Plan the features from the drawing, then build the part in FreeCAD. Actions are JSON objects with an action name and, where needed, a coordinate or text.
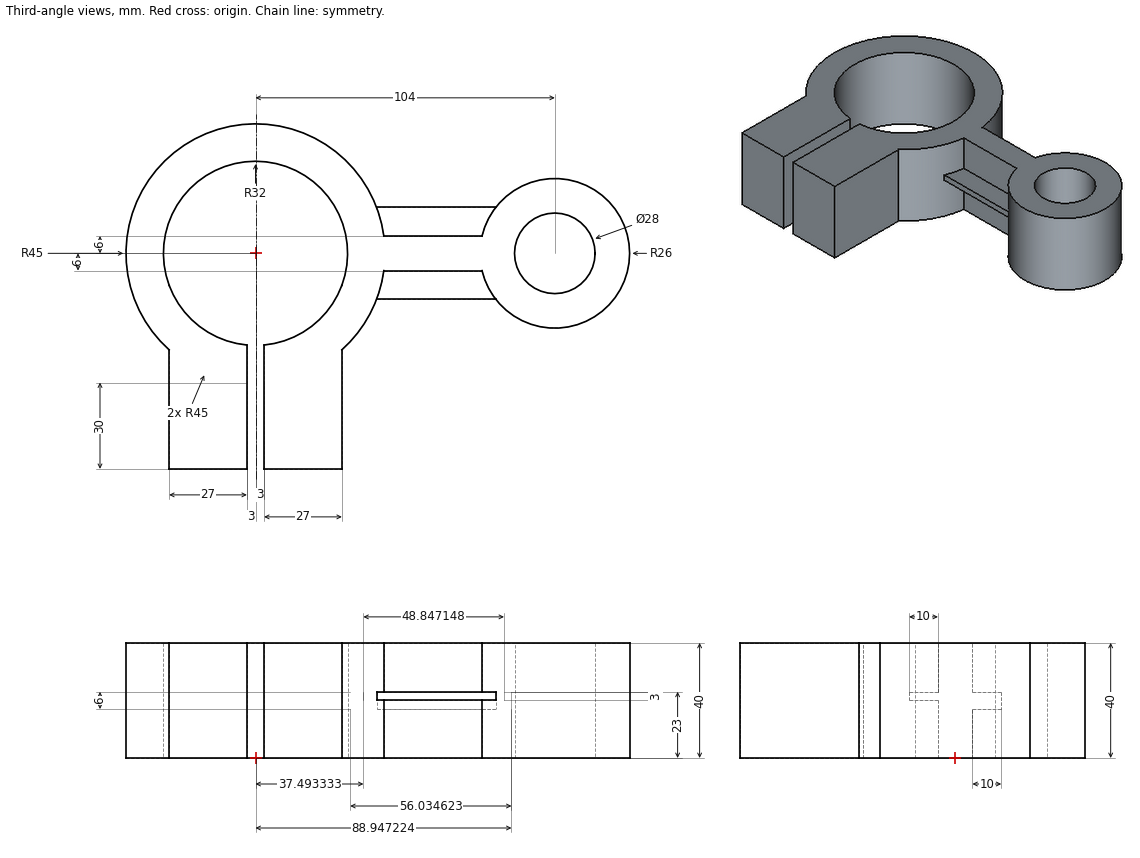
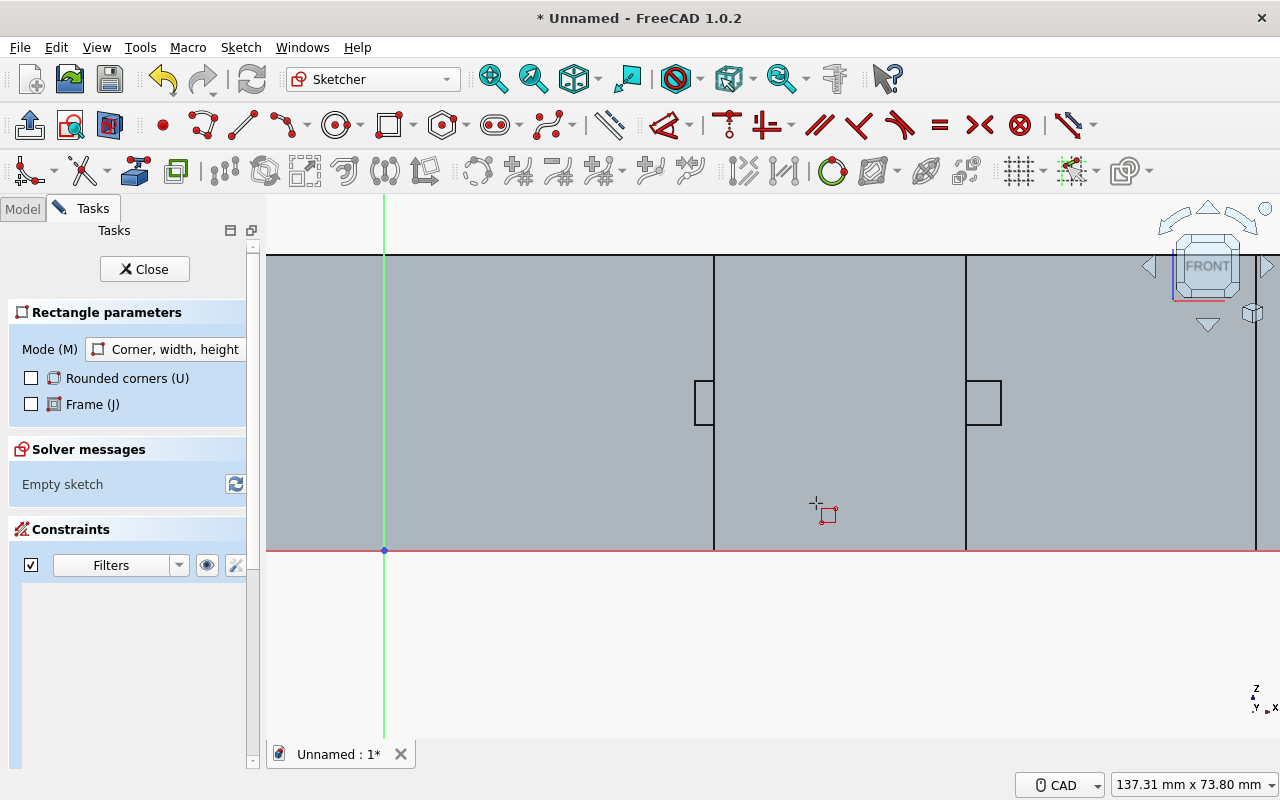
{"action": "left_click", "coordinate": [661, 381]}
{"action": "mouse_move", "coordinate": [1022, 403]}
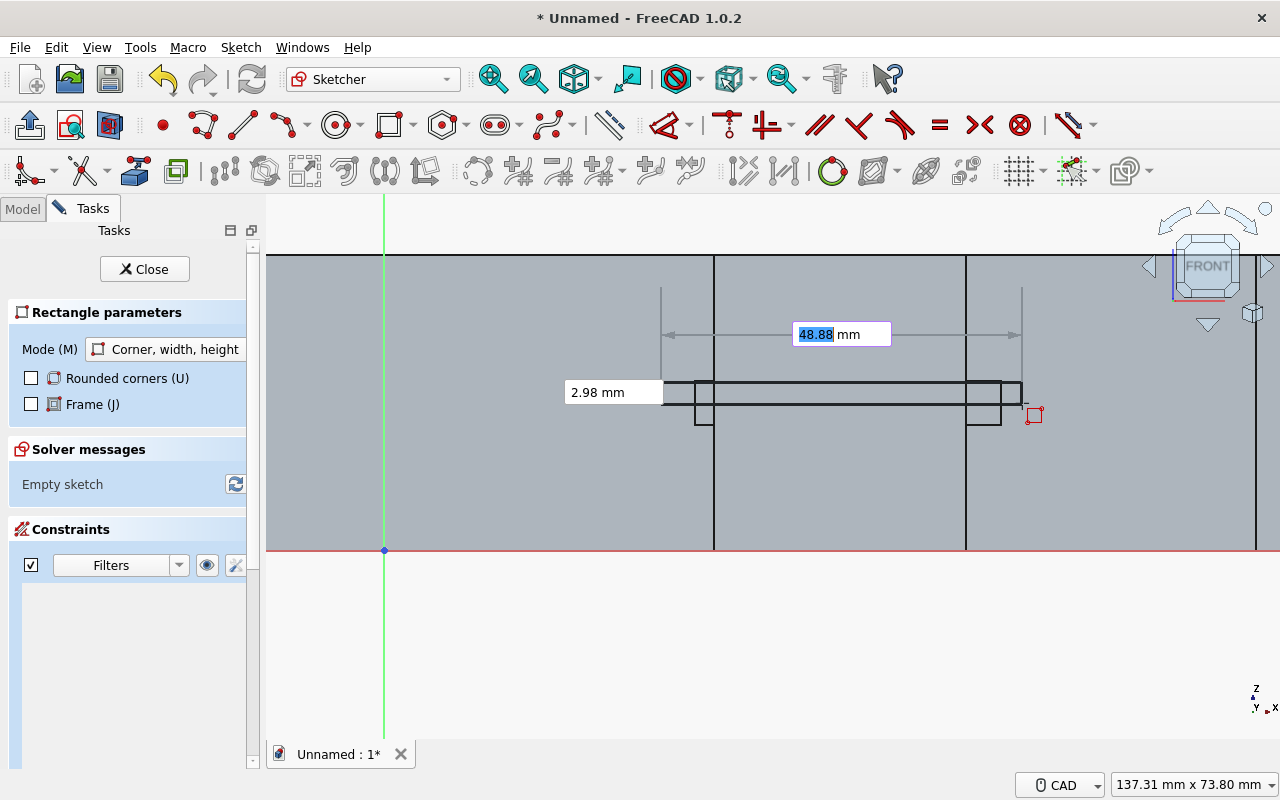
{"action": "type", "text": "48.847148"}
{"action": "key", "text": "Tab"}
{"action": "type", "text": "3"}
{"action": "key", "text": "Return"}
{"action": "key", "text": "Escape"}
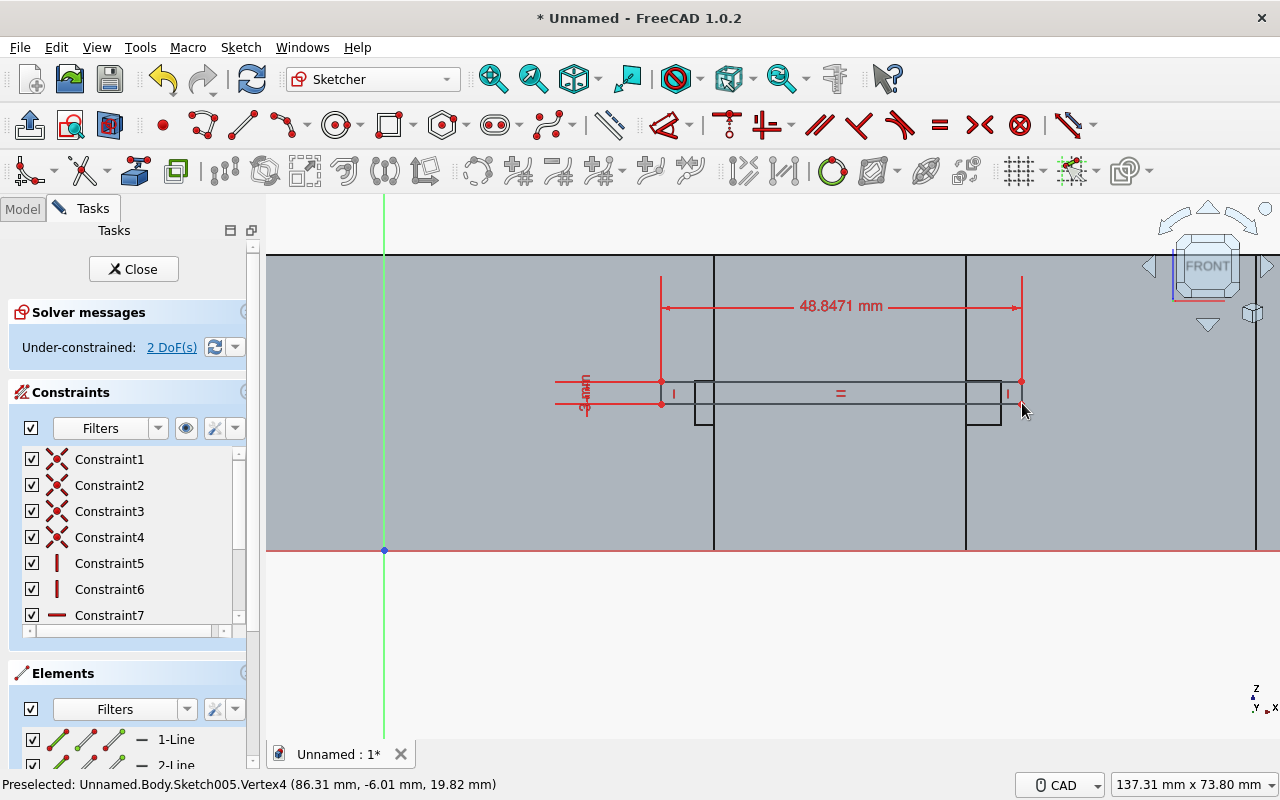
{"action": "key", "text": "d"}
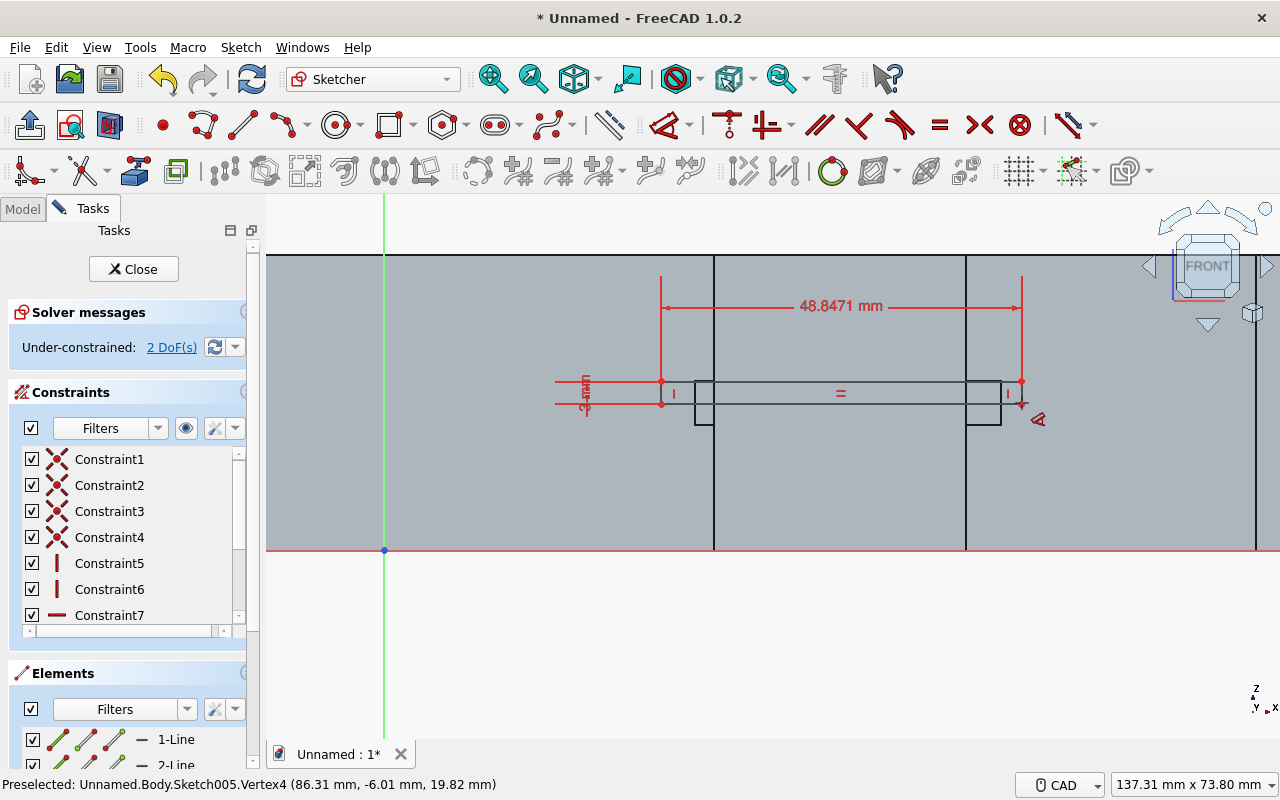
{"action": "left_click", "coordinate": [661, 382]}
{"action": "left_click", "coordinate": [350, 466]}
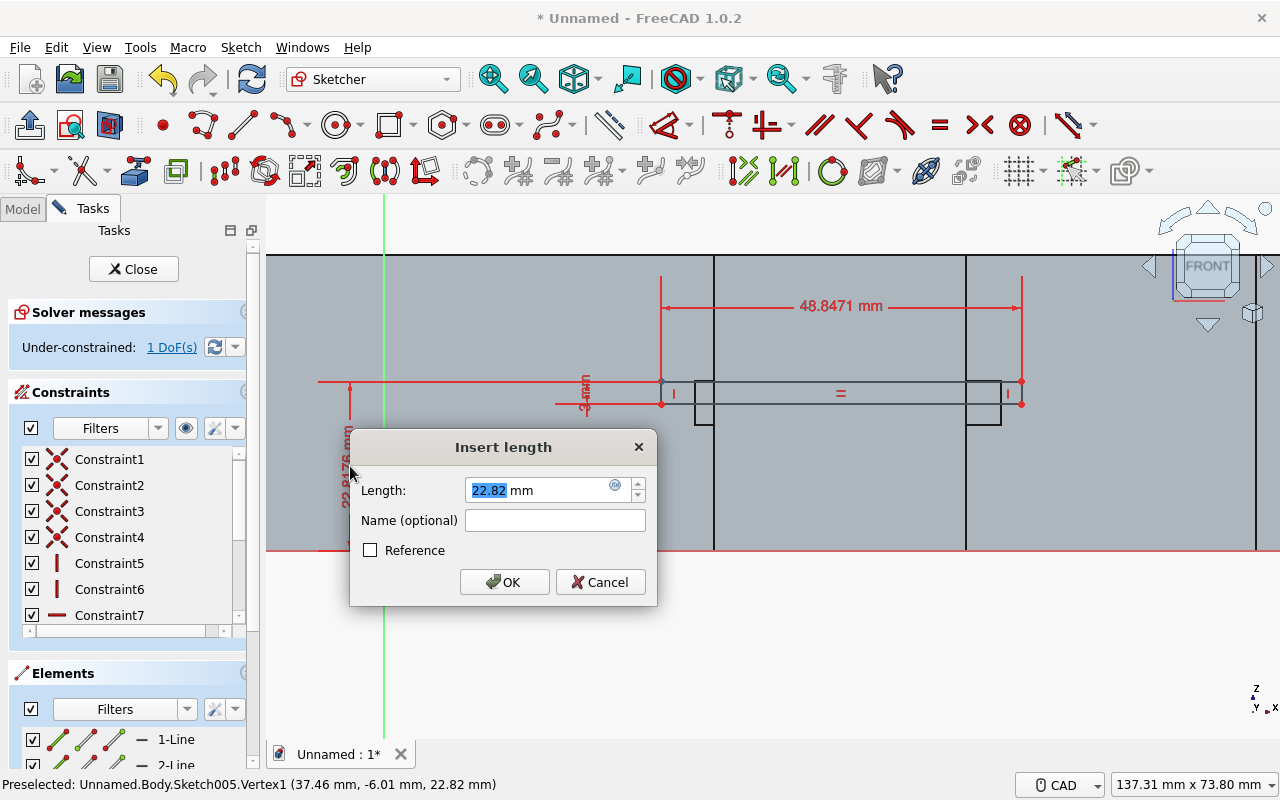
{"action": "type", "text": "23"}
{"action": "key", "text": "Return"}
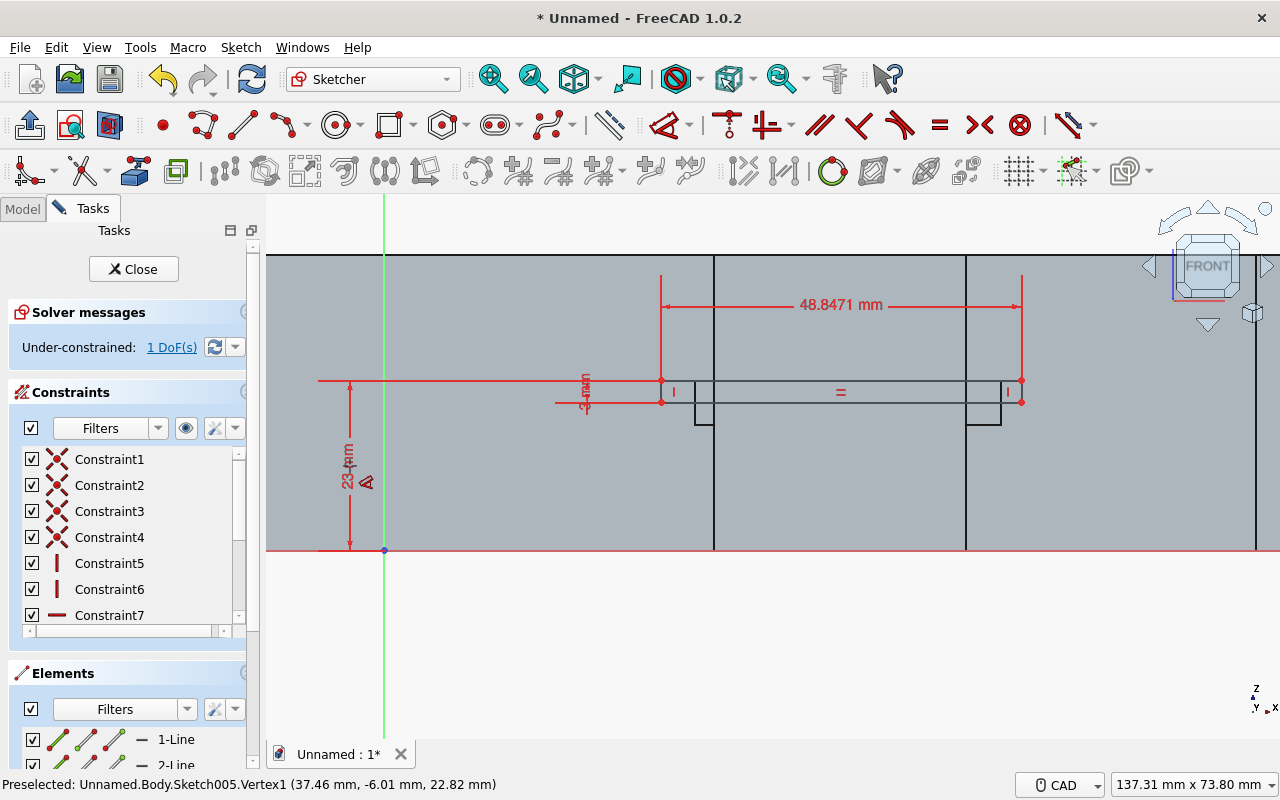
{"action": "left_click", "coordinate": [661, 381]}
{"action": "left_click", "coordinate": [523, 585]}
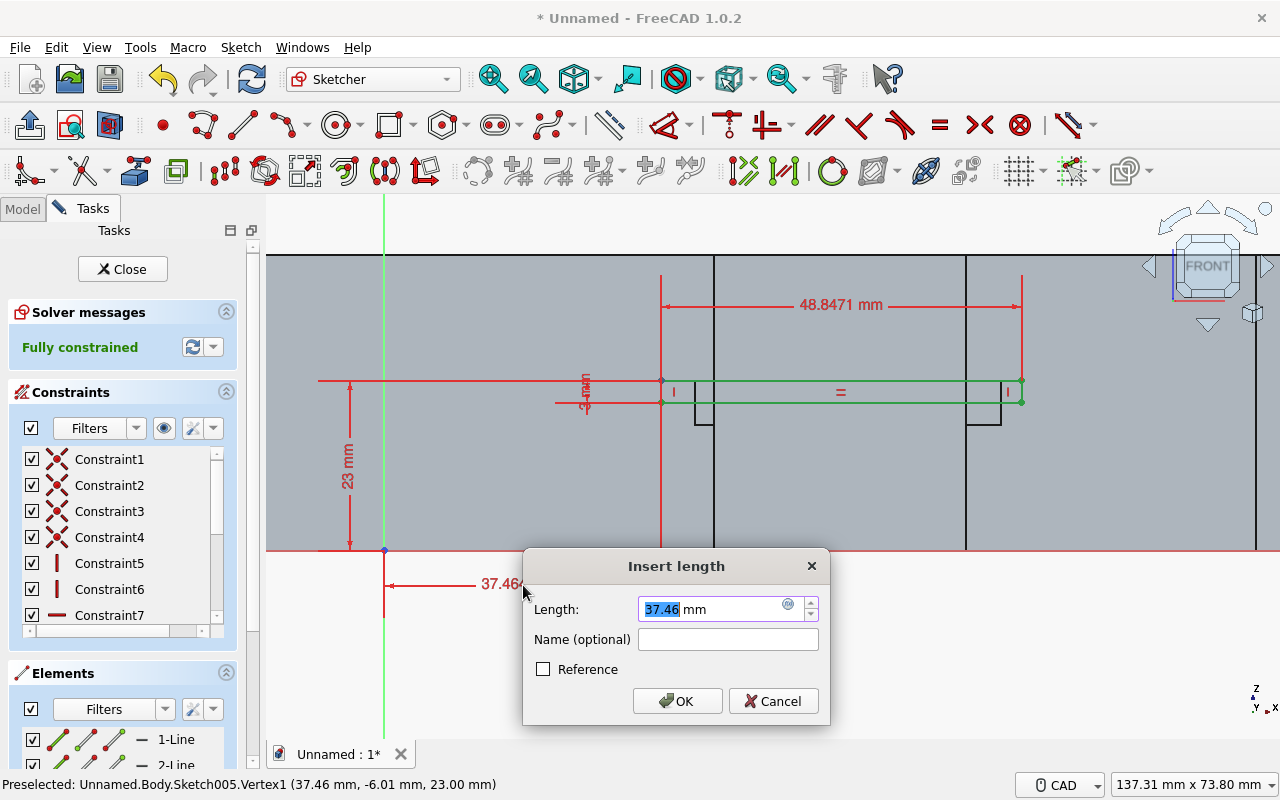
{"action": "type", "text": "37.493333"}
{"action": "key", "text": "Return"}
{"action": "key", "text": "Escape"}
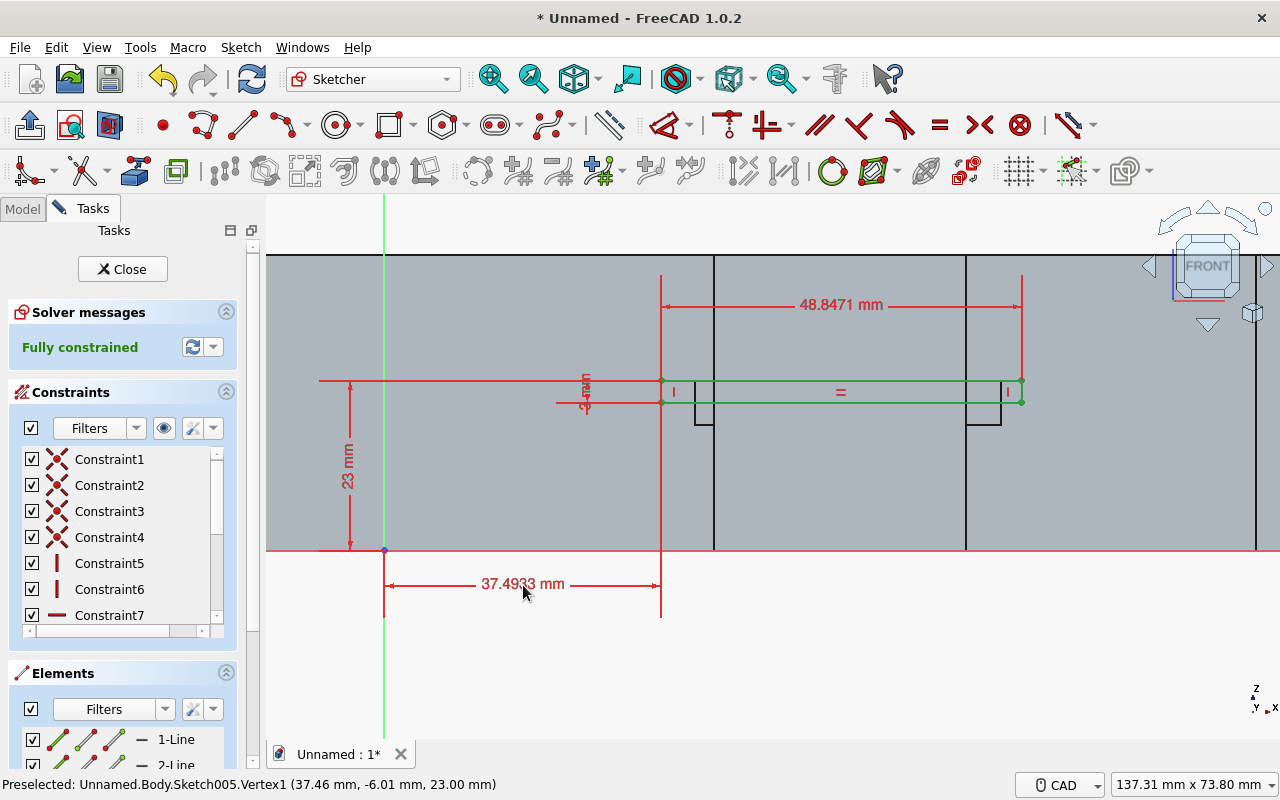
{"action": "left_click", "coordinate": [123, 269]}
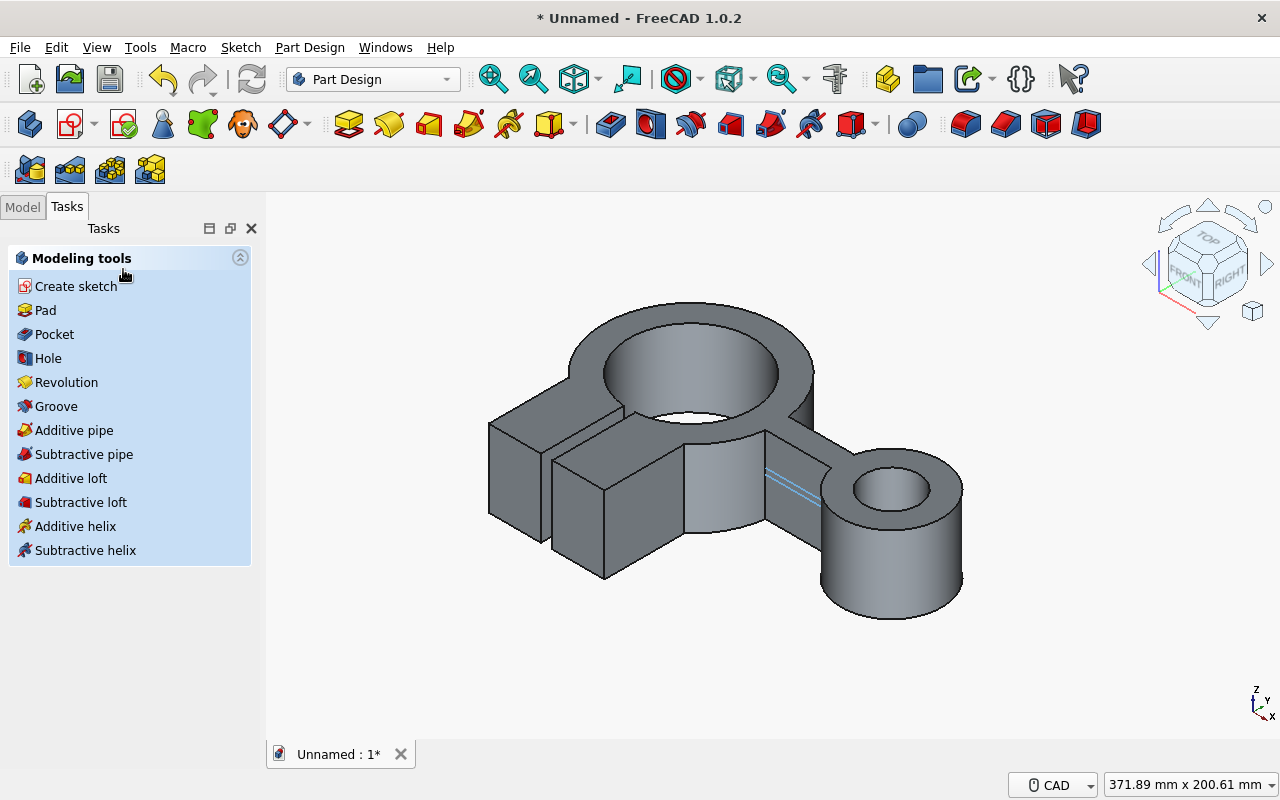
{"action": "left_click", "coordinate": [350, 124]}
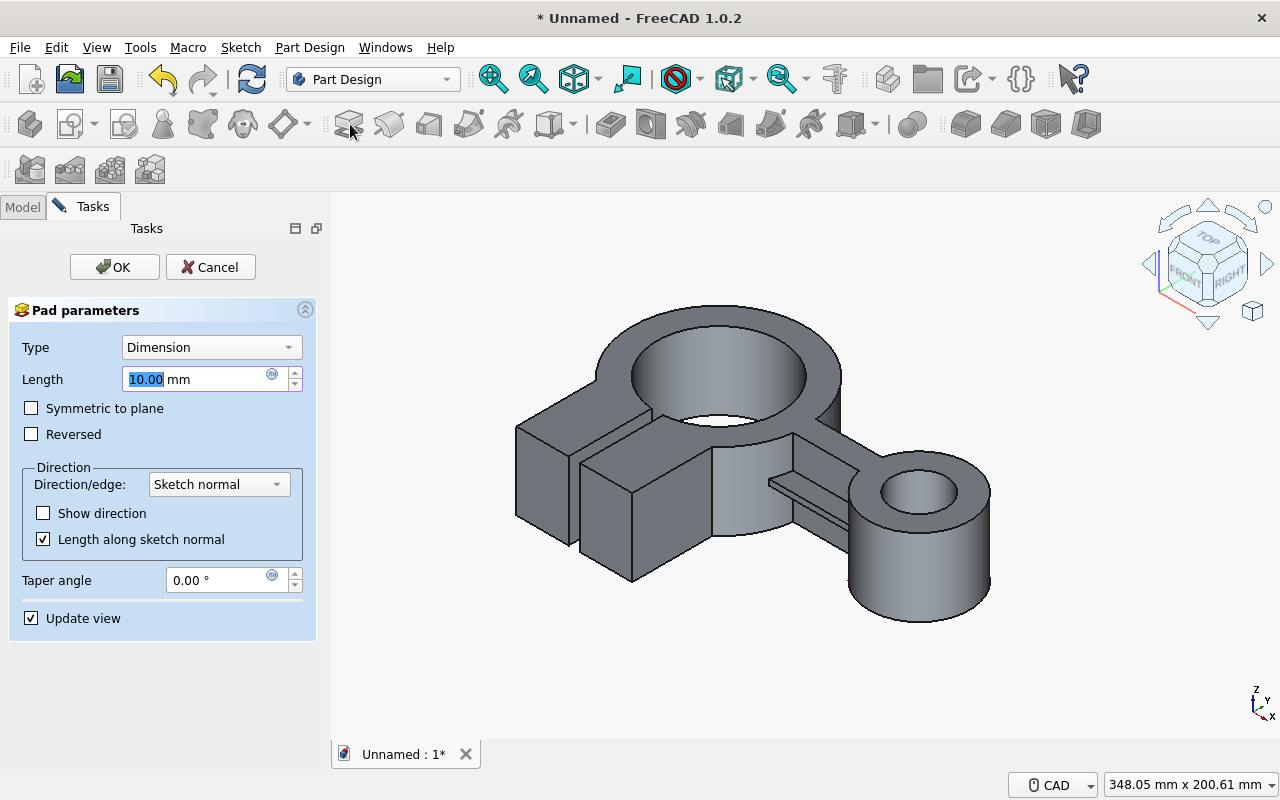
{"action": "type", "text": "10"}
{"action": "key", "text": "Tab"}